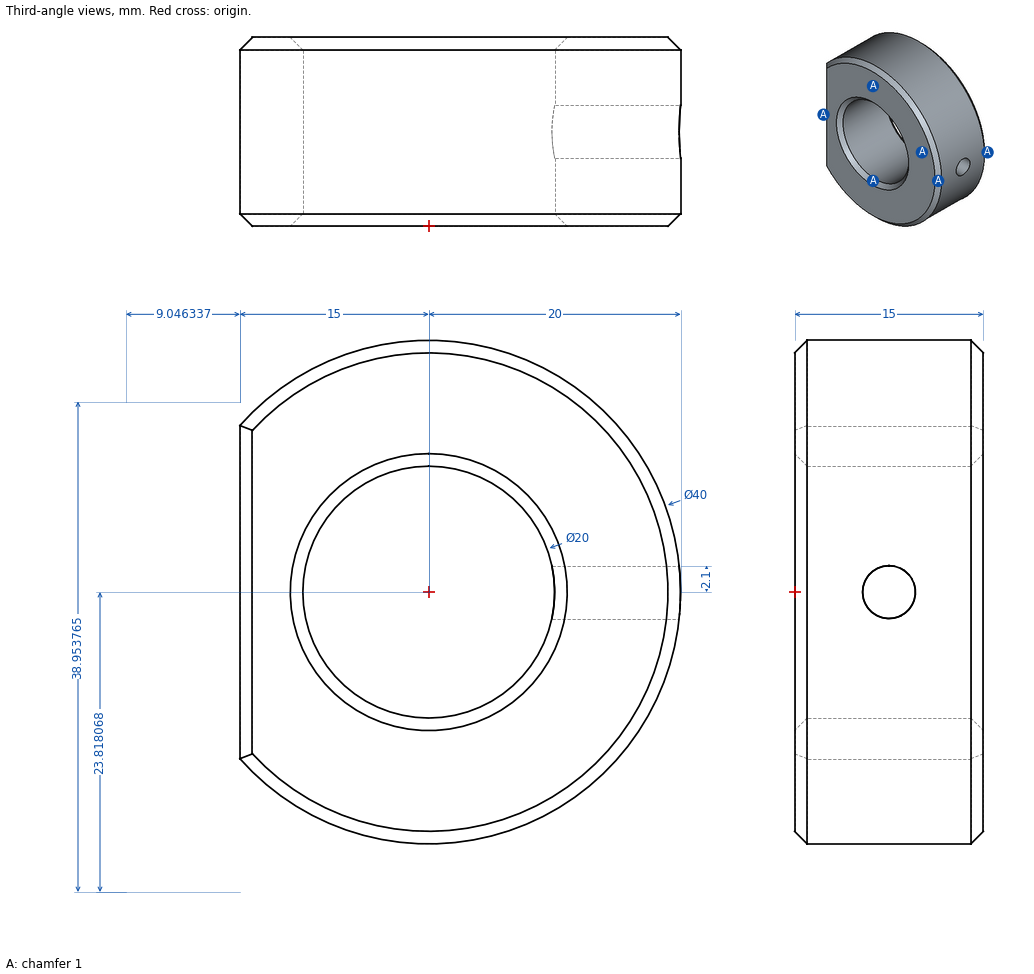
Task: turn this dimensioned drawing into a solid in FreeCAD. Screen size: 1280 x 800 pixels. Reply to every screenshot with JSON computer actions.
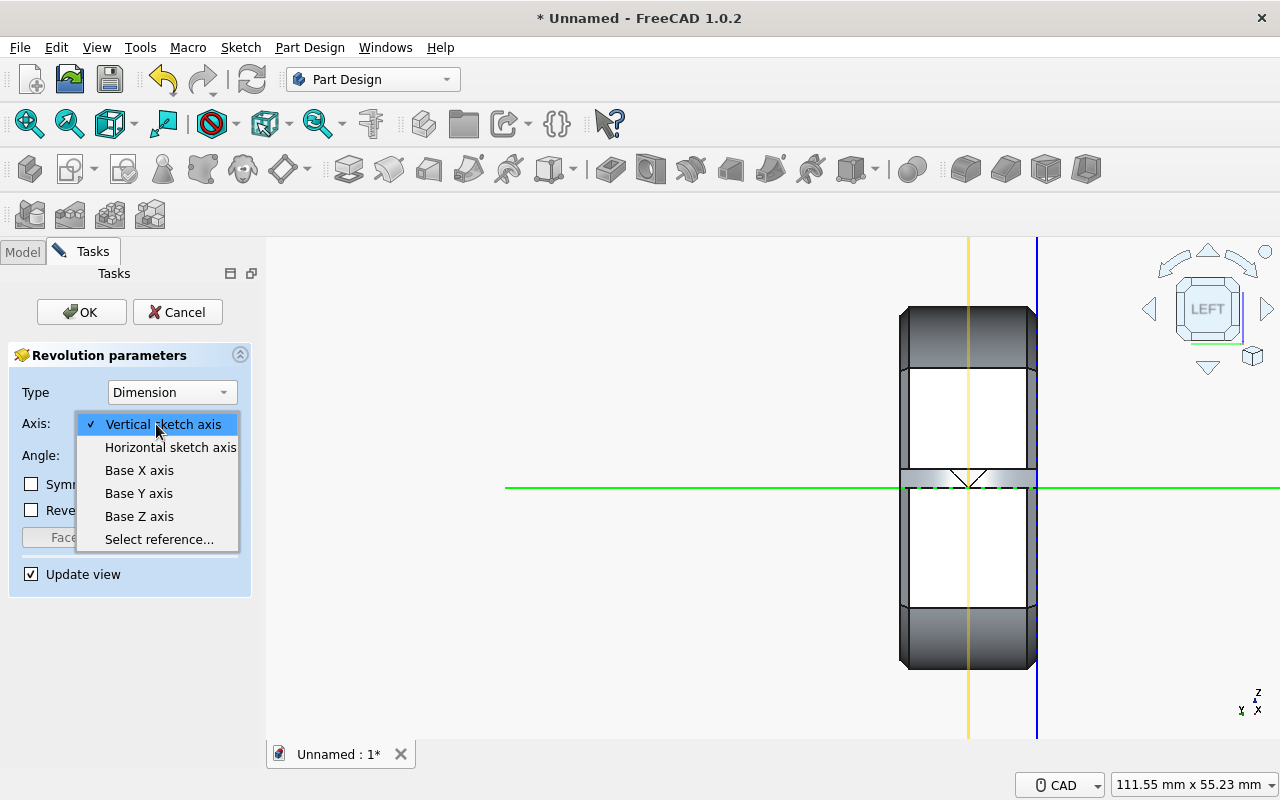
{"action": "left_click", "coordinate": [156, 448]}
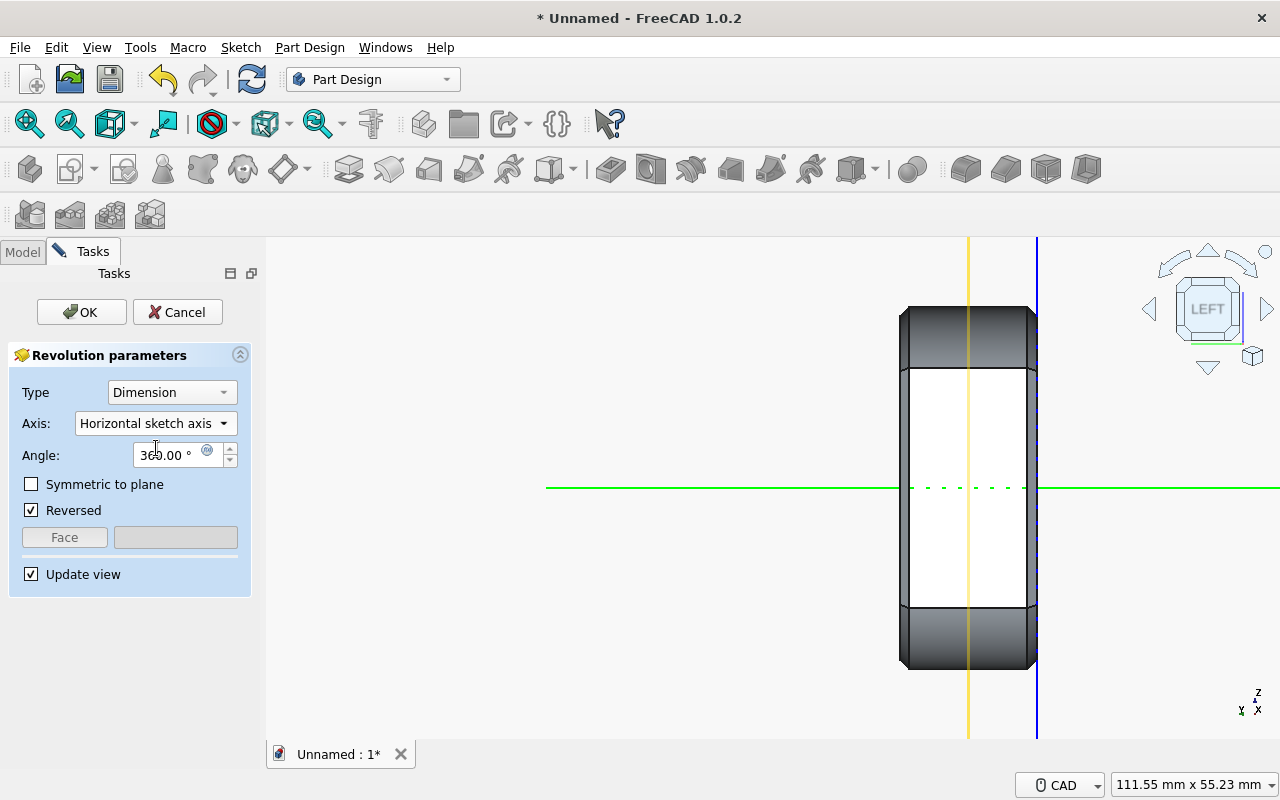
{"action": "left_click", "coordinate": [82, 312]}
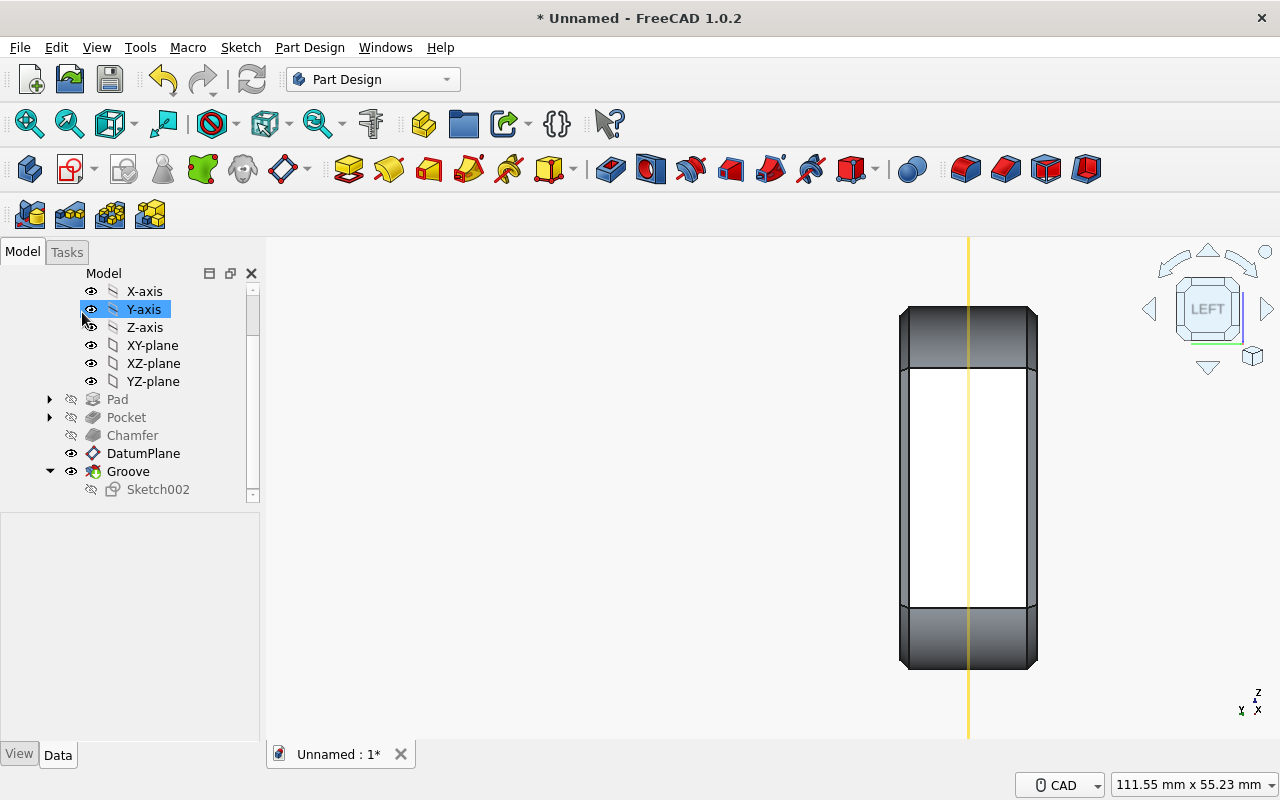
{"action": "left_click", "coordinate": [116, 453]}
{"action": "key", "text": "space"}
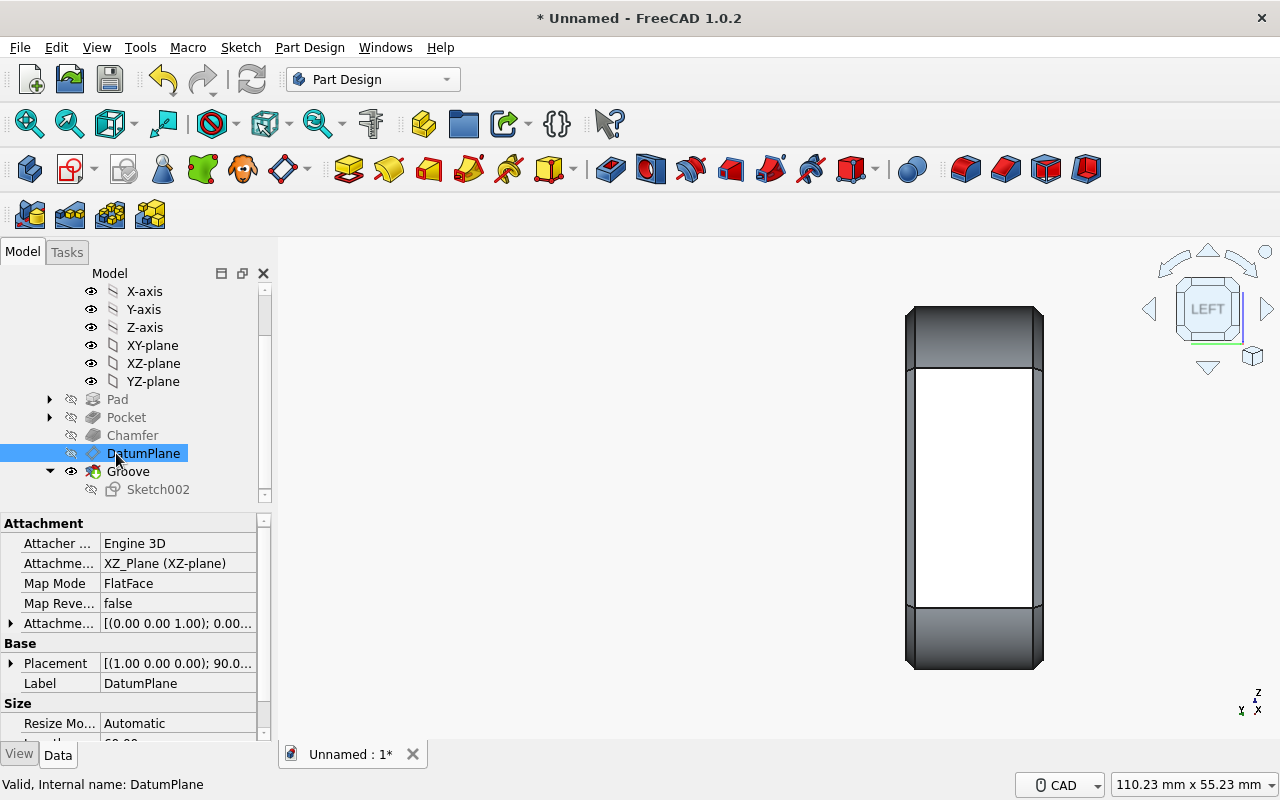
{"action": "key", "text": "0"}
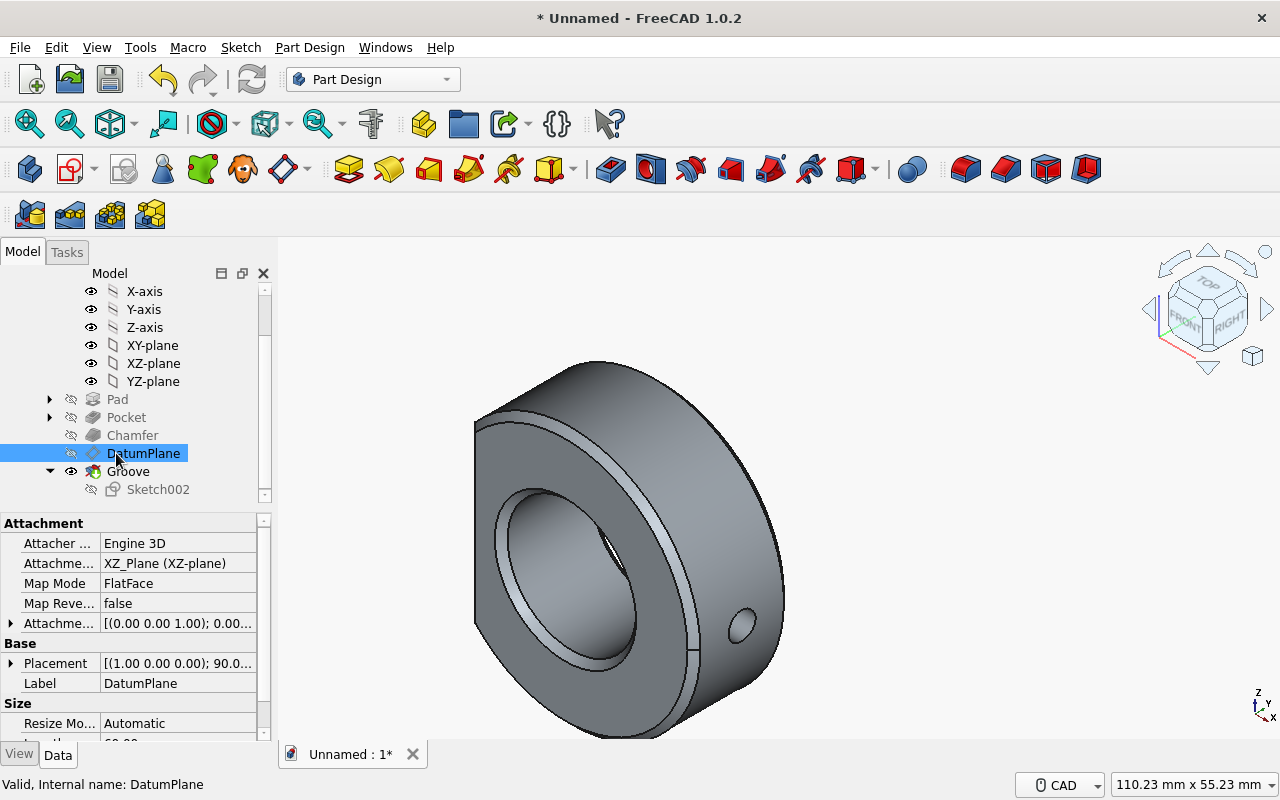
{"action": "key", "text": "v f"}